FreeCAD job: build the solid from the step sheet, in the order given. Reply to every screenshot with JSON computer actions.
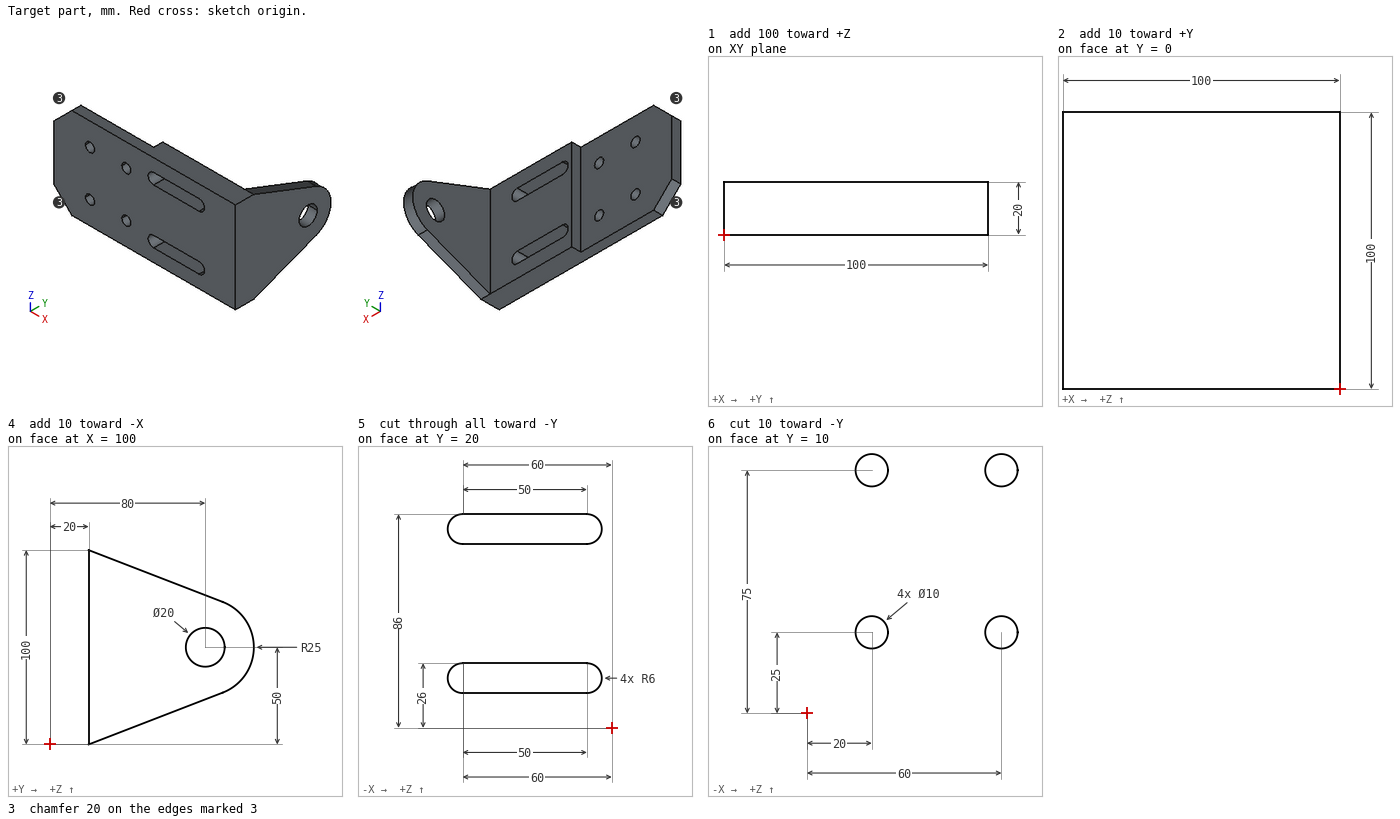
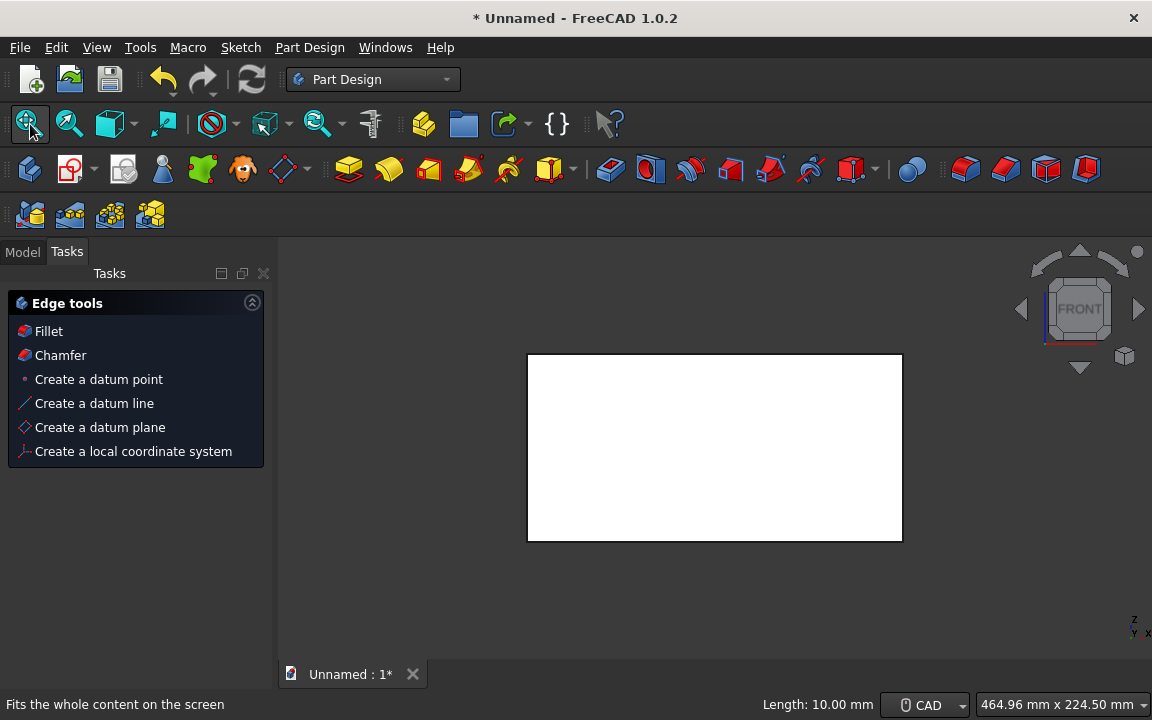
{"action": "key", "text": "3"}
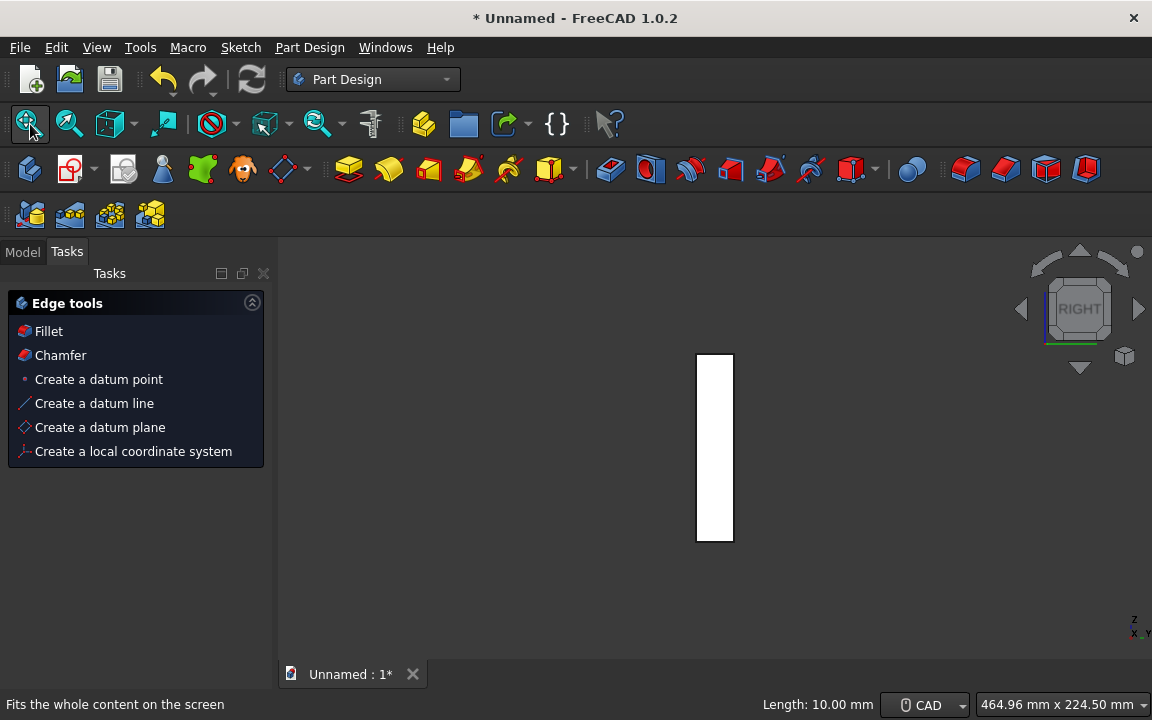
{"action": "left_click", "coordinate": [30, 124]}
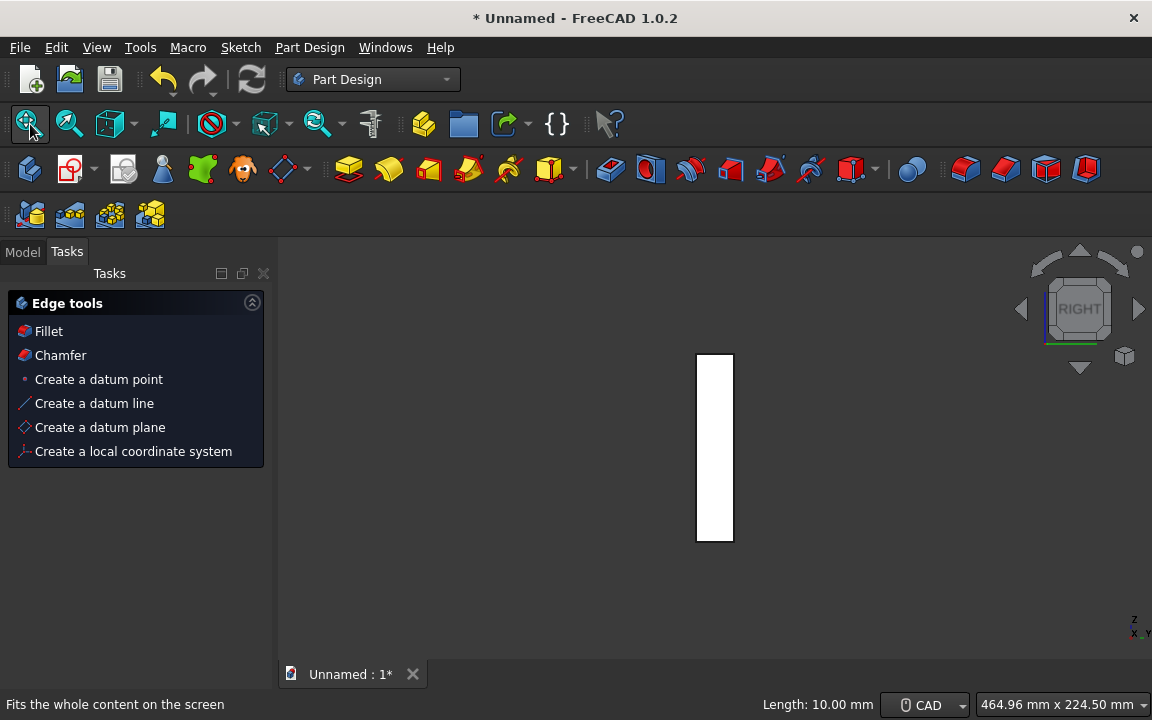
{"action": "scroll", "coordinate": [706, 541], "scroll_direction": "up", "scroll_amount": 4}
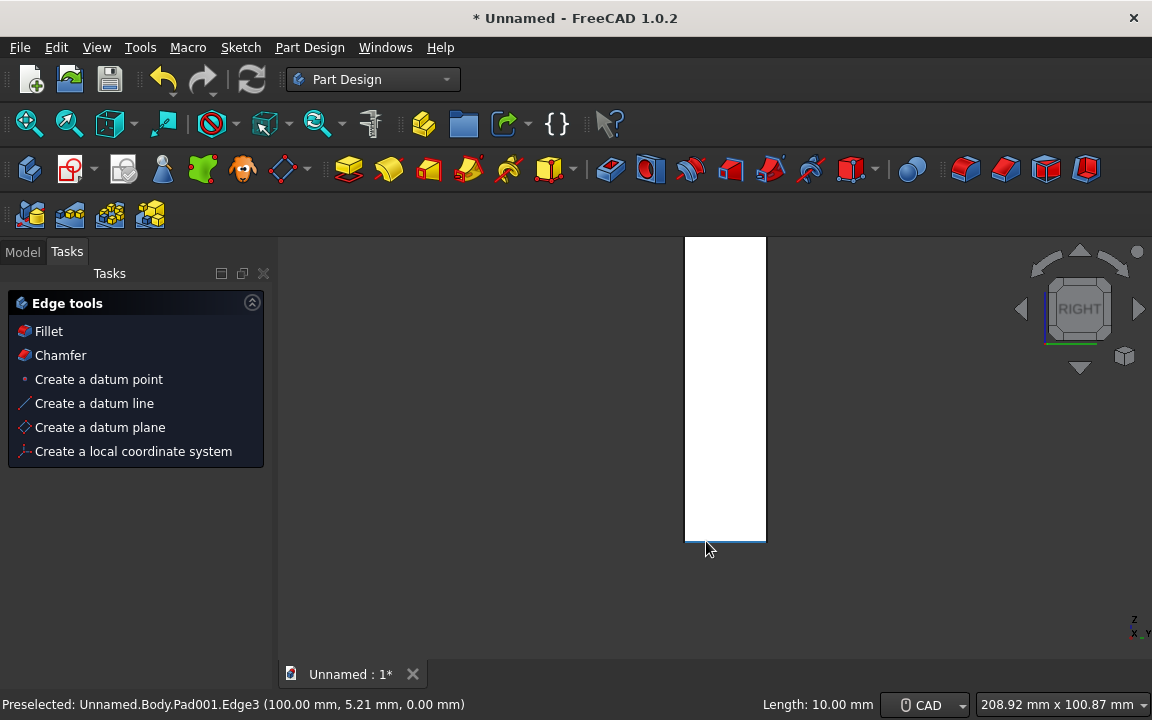
{"action": "left_click", "coordinate": [30, 124]}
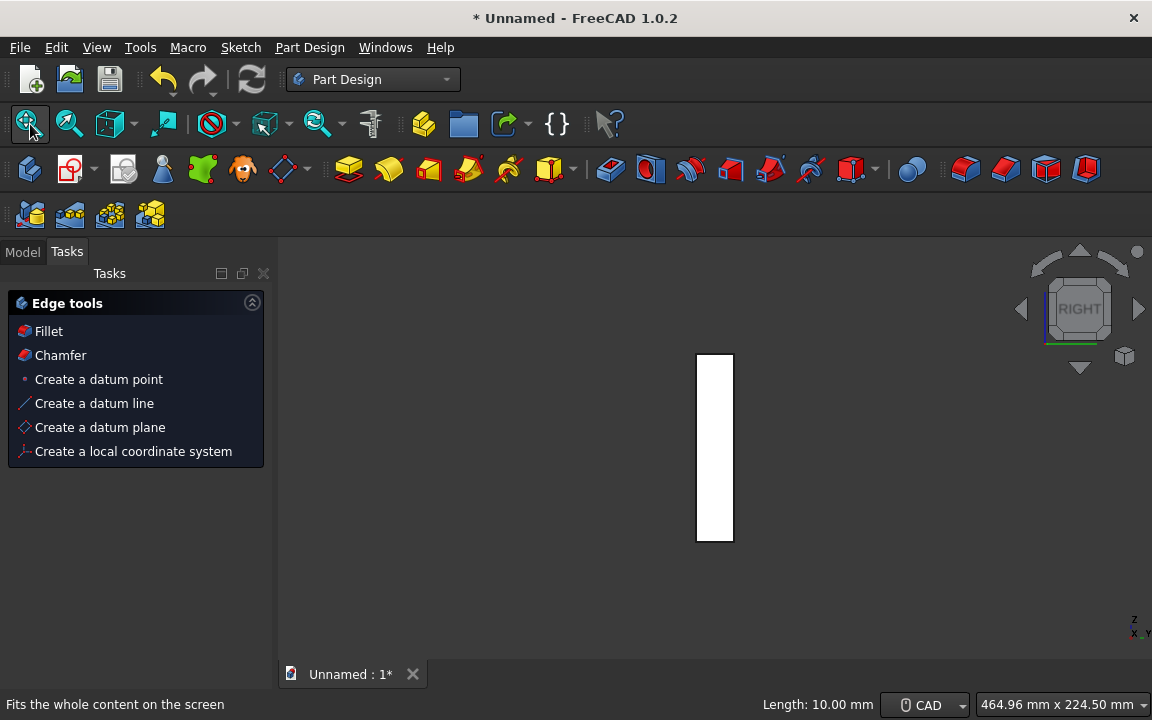
{"action": "key", "text": "5"}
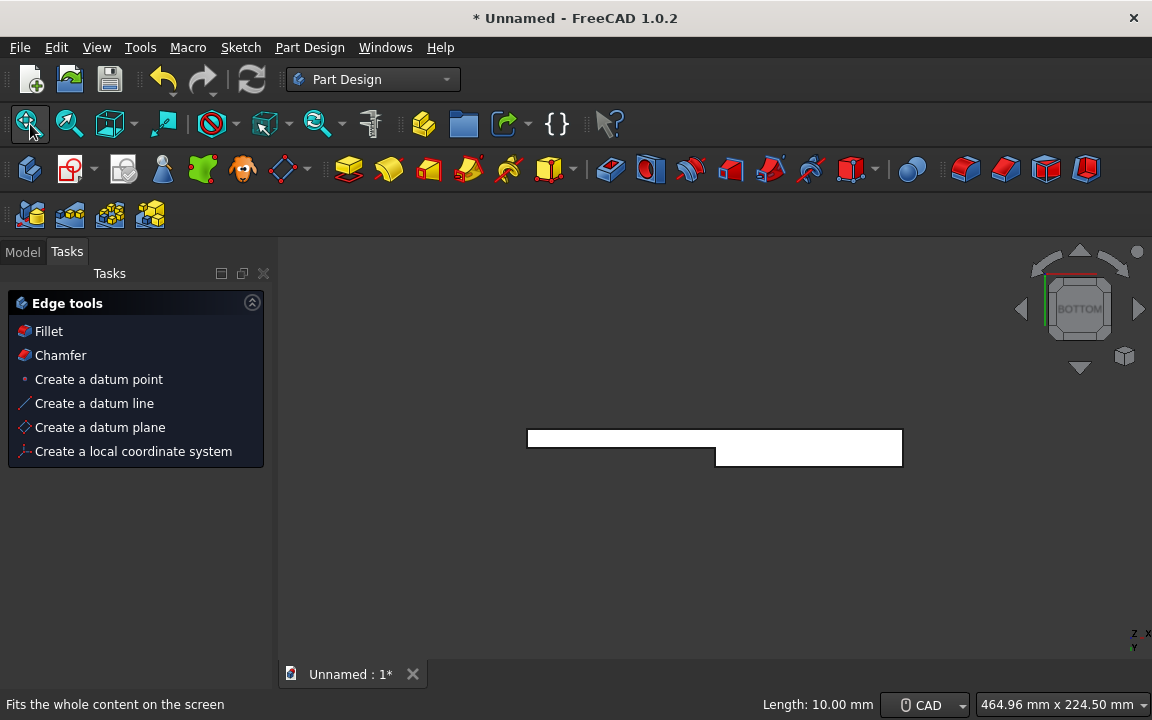
{"action": "left_click", "coordinate": [30, 124]}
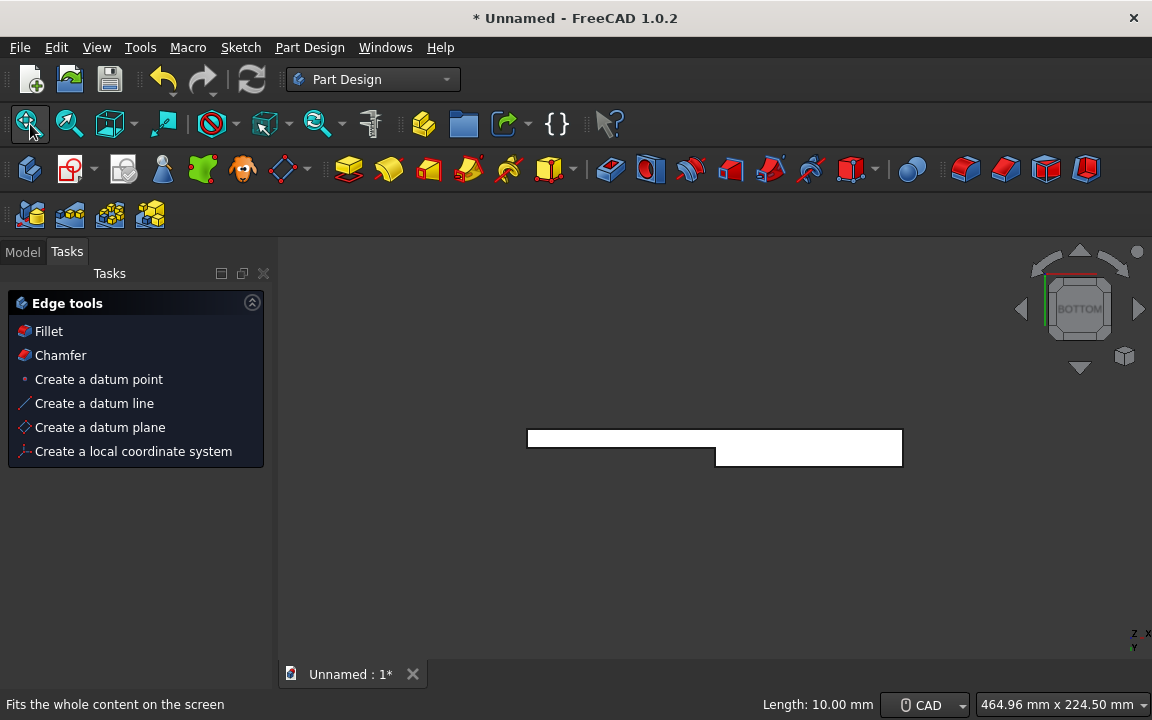
{"action": "left_click", "coordinate": [527, 438], "text": "ctrl"}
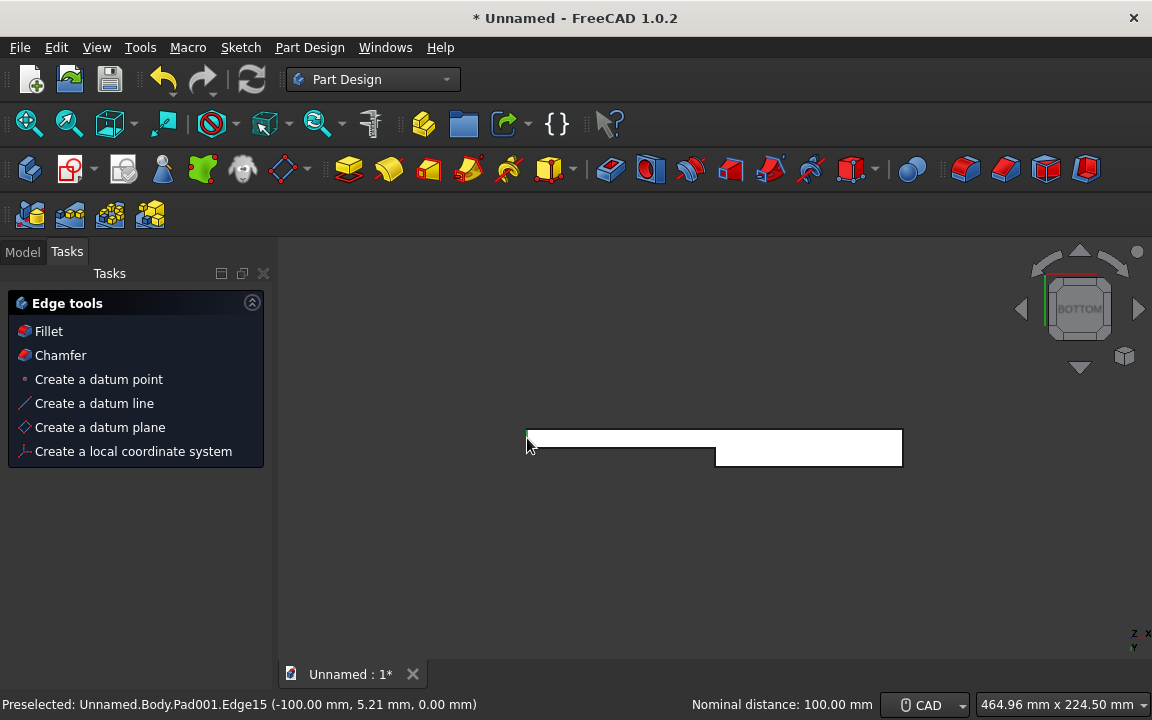
{"action": "left_click", "coordinate": [1006, 170]}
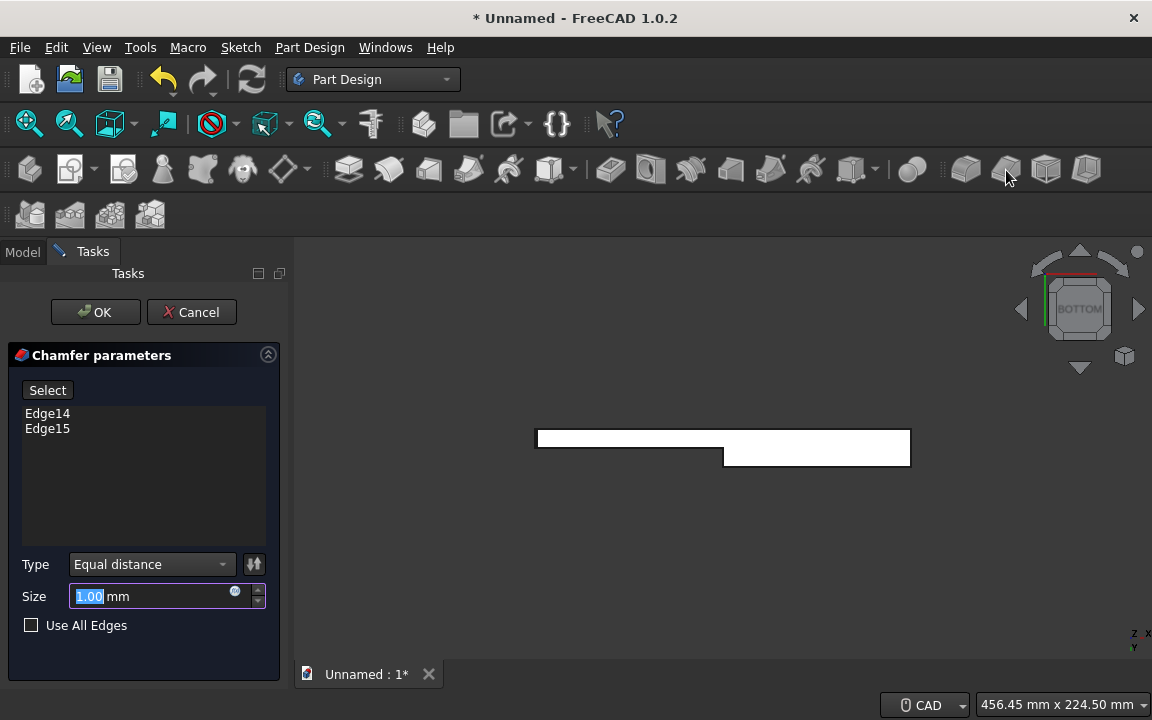
{"action": "type", "text": "20"}
{"action": "key", "text": "Tab"}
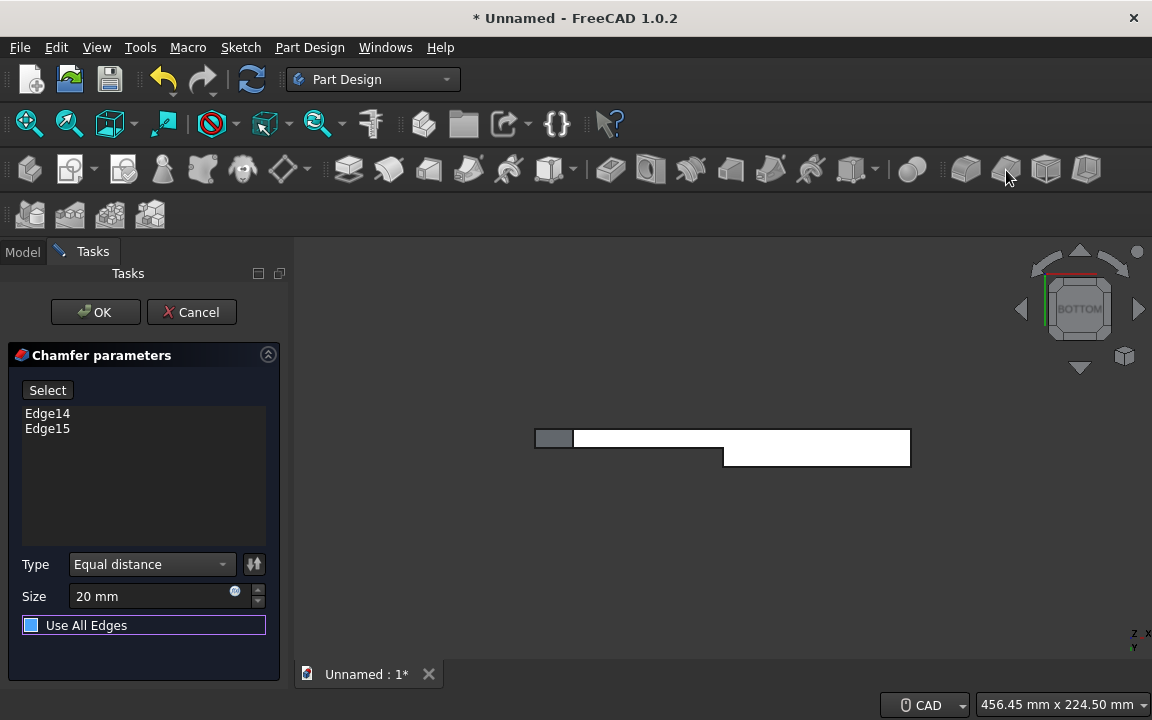
{"action": "left_click", "coordinate": [96, 312]}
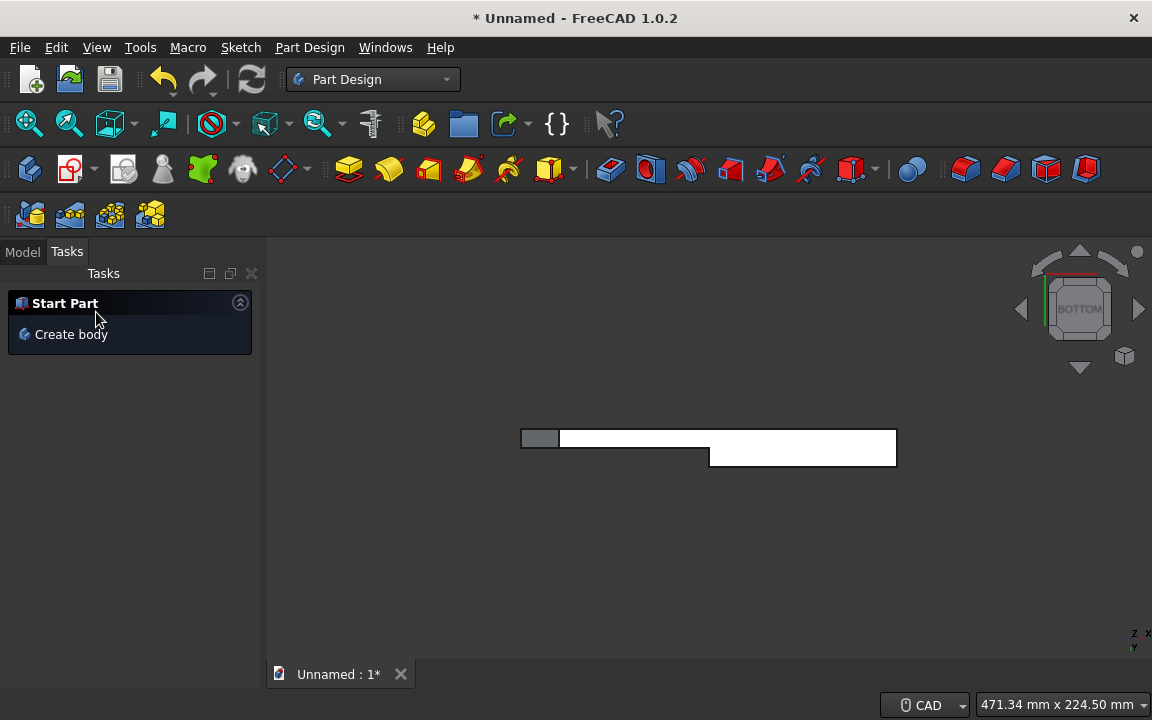
{"action": "left_click", "coordinate": [30, 124]}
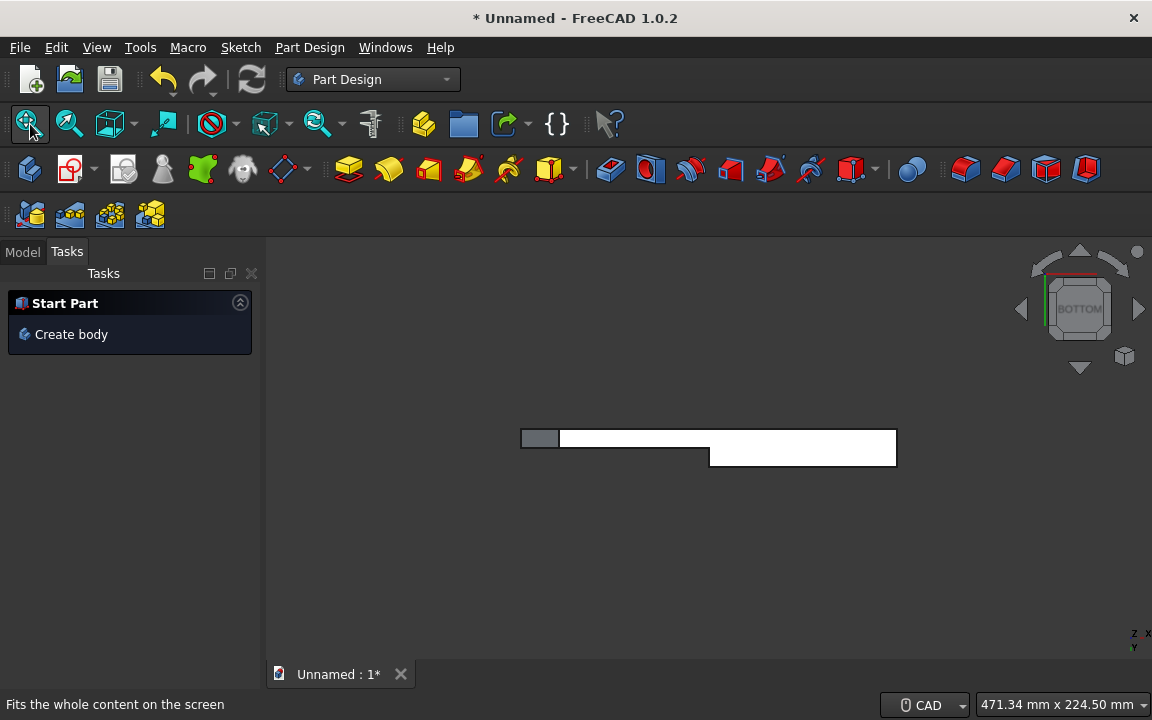
{"action": "key", "text": "0"}